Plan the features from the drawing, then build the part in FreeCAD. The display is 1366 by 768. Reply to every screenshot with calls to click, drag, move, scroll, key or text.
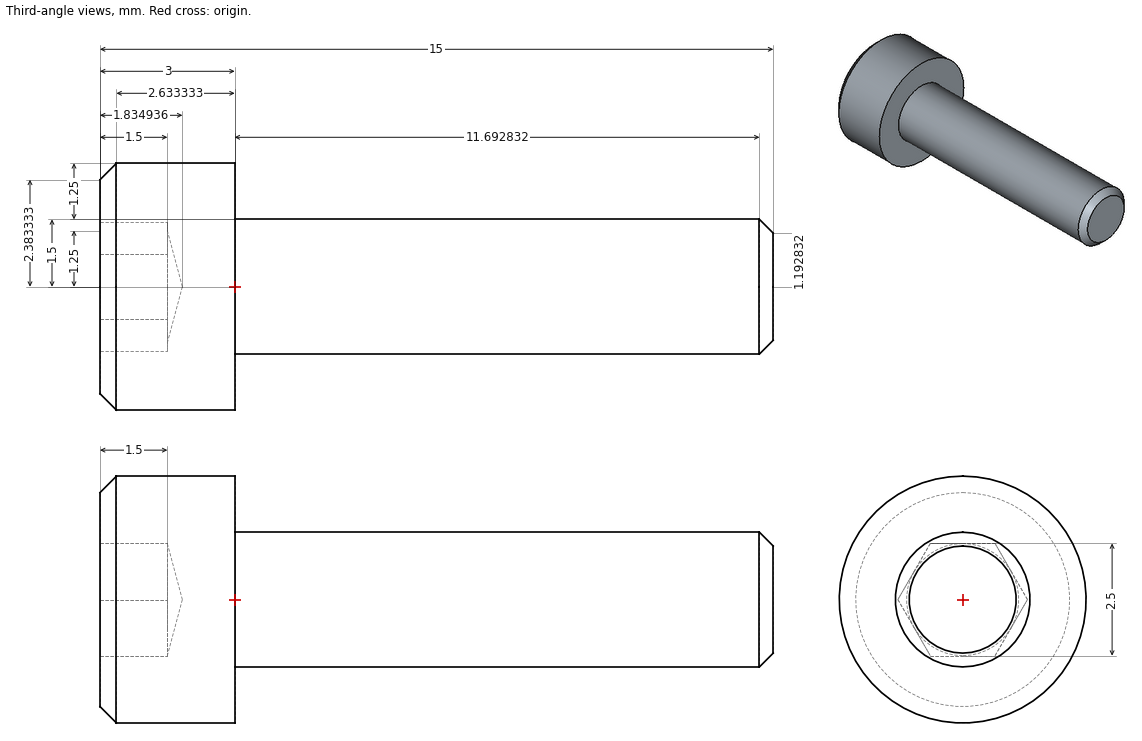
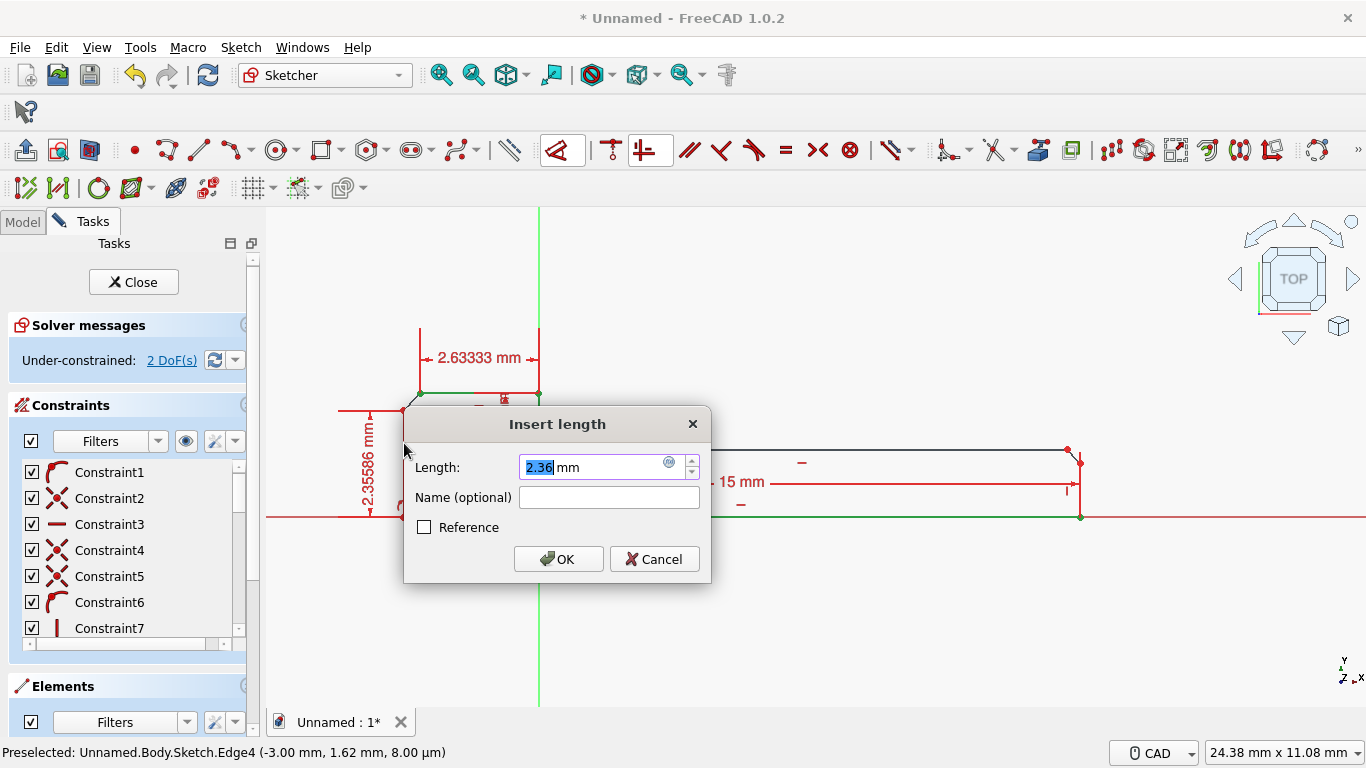
text(2.383333)
key(Return)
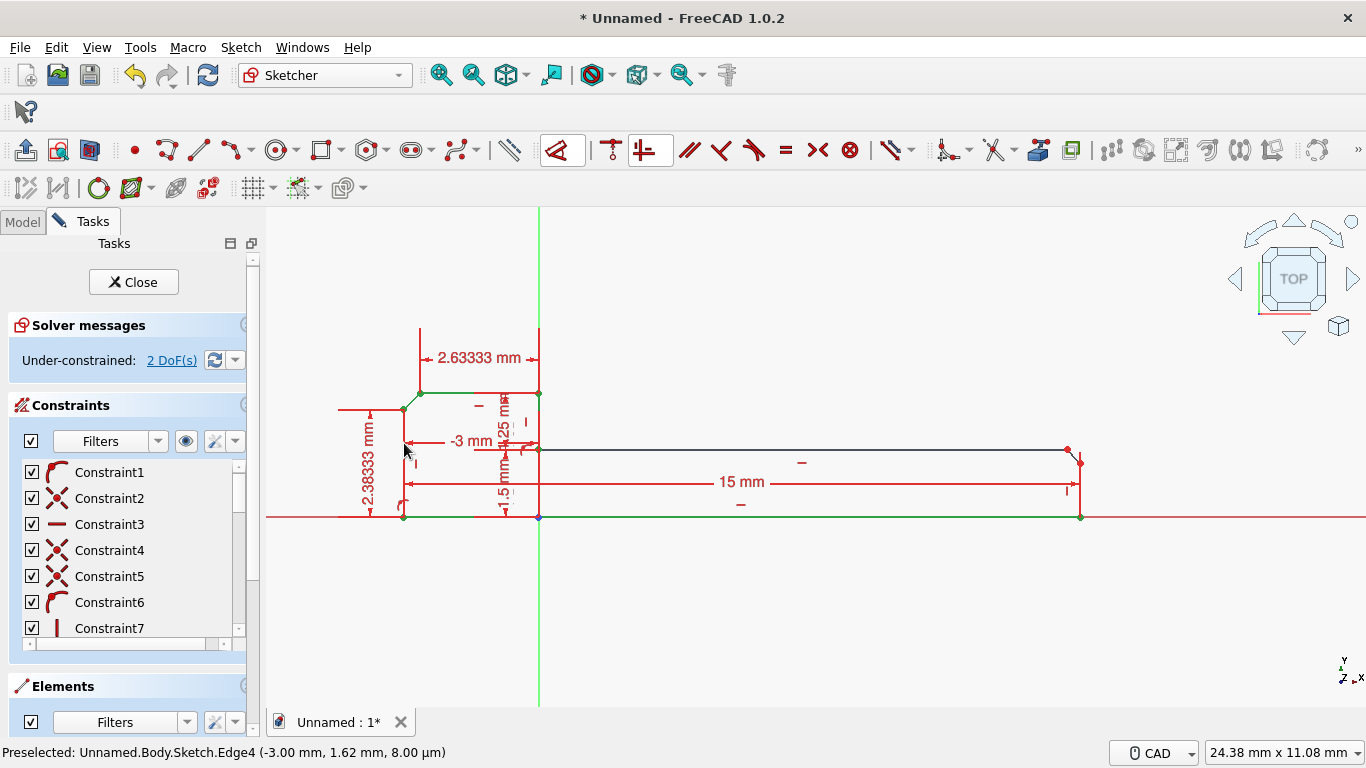
click(1080, 501)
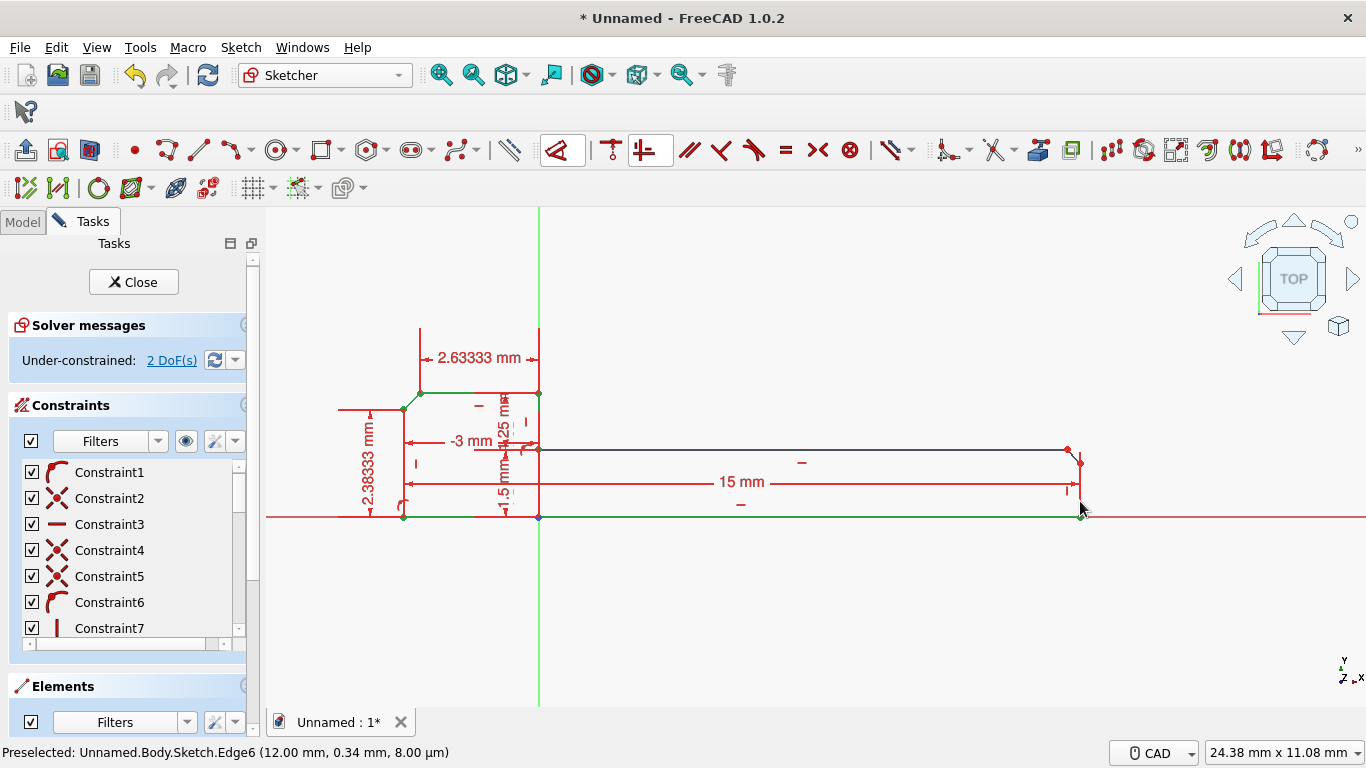
click(580, 150)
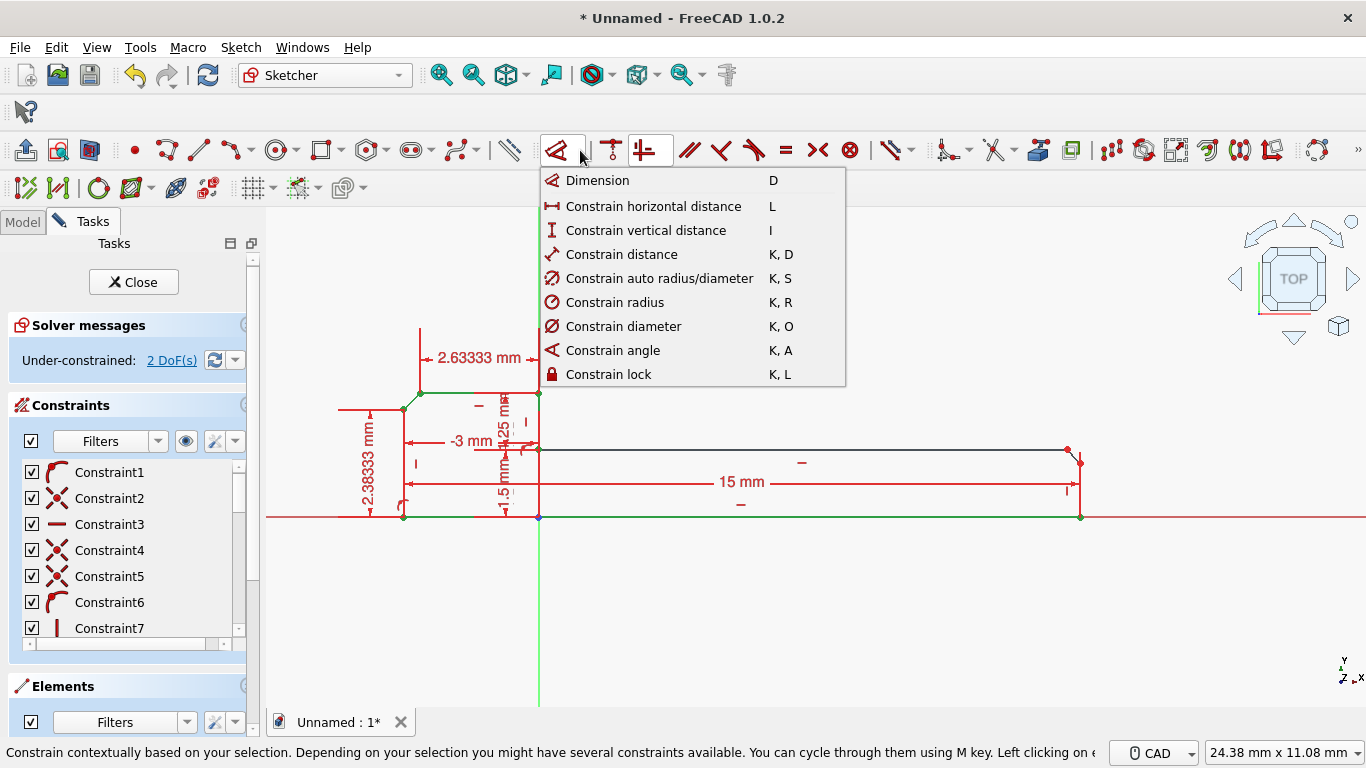
click(693, 230)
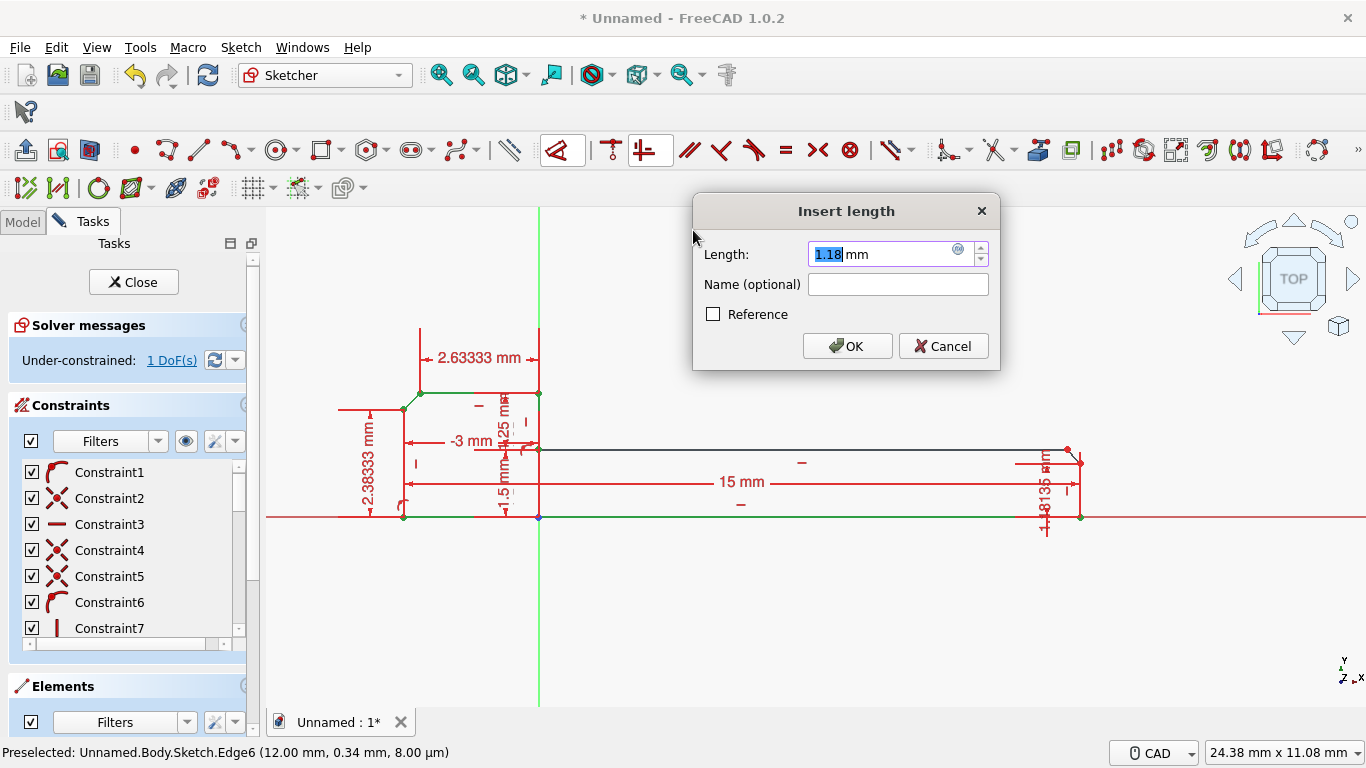
text(1.192832)
key(Return)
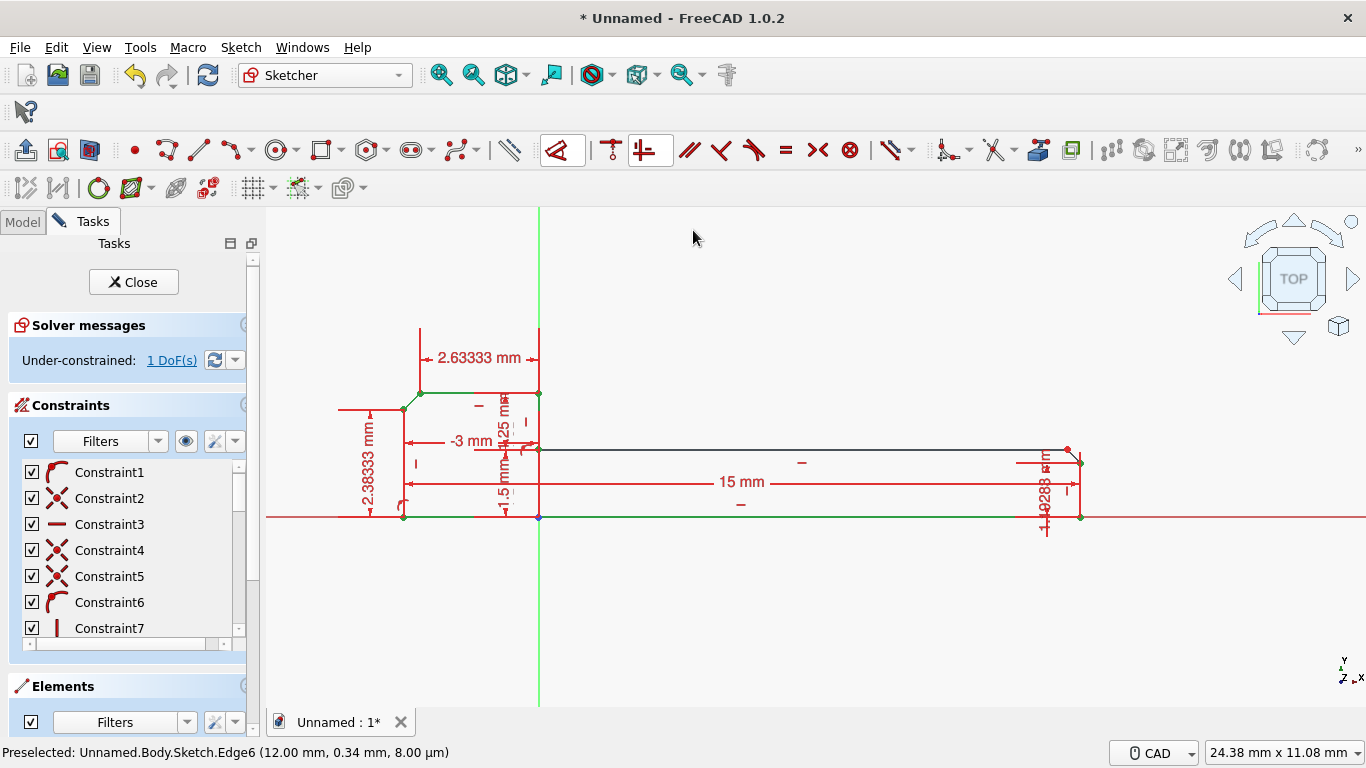
click(909, 450)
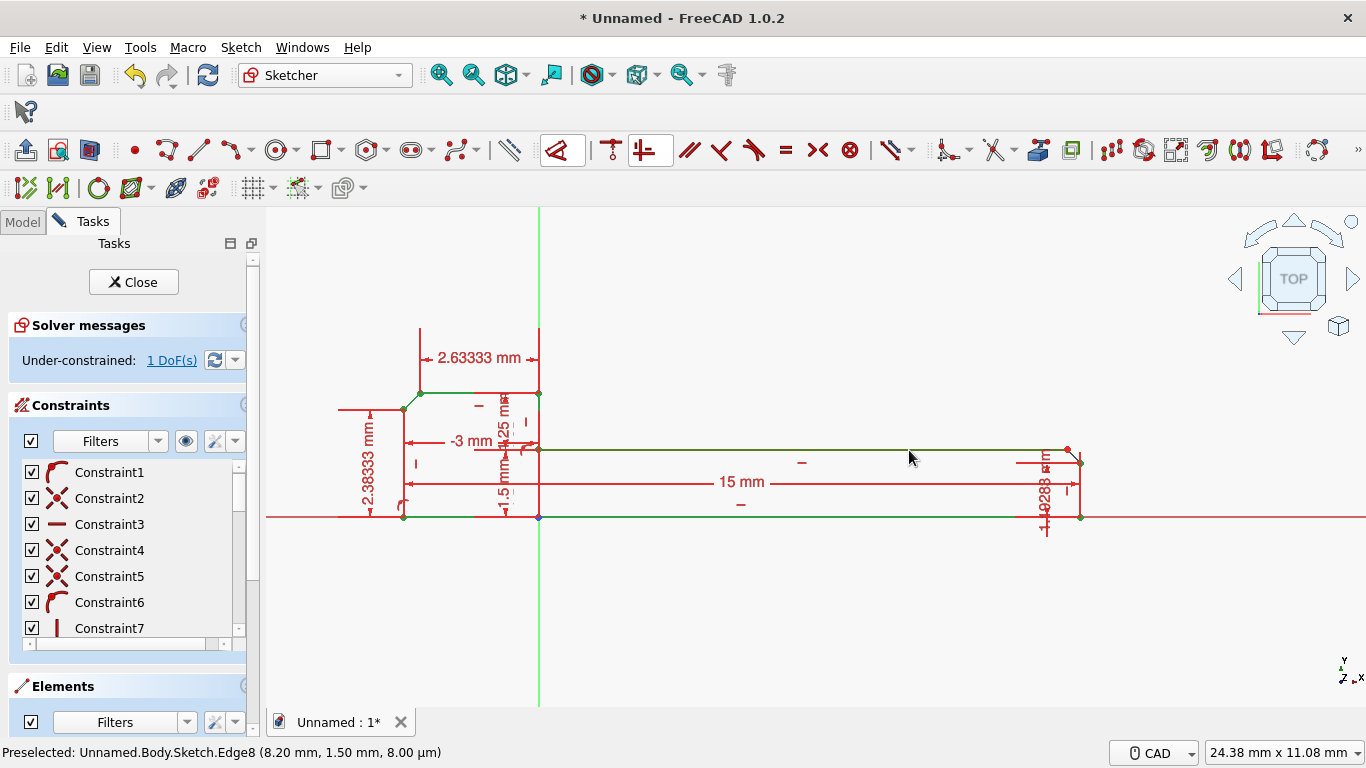
click(580, 150)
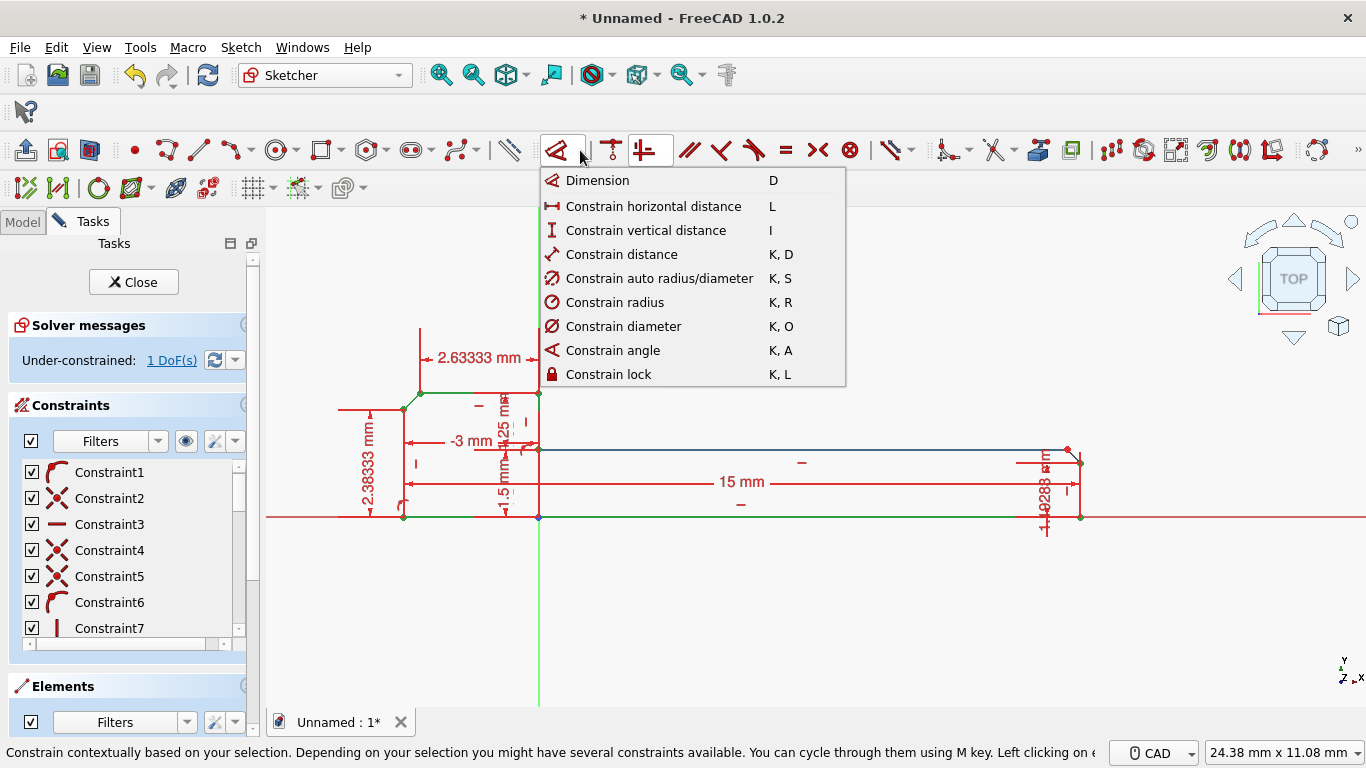
click(693, 206)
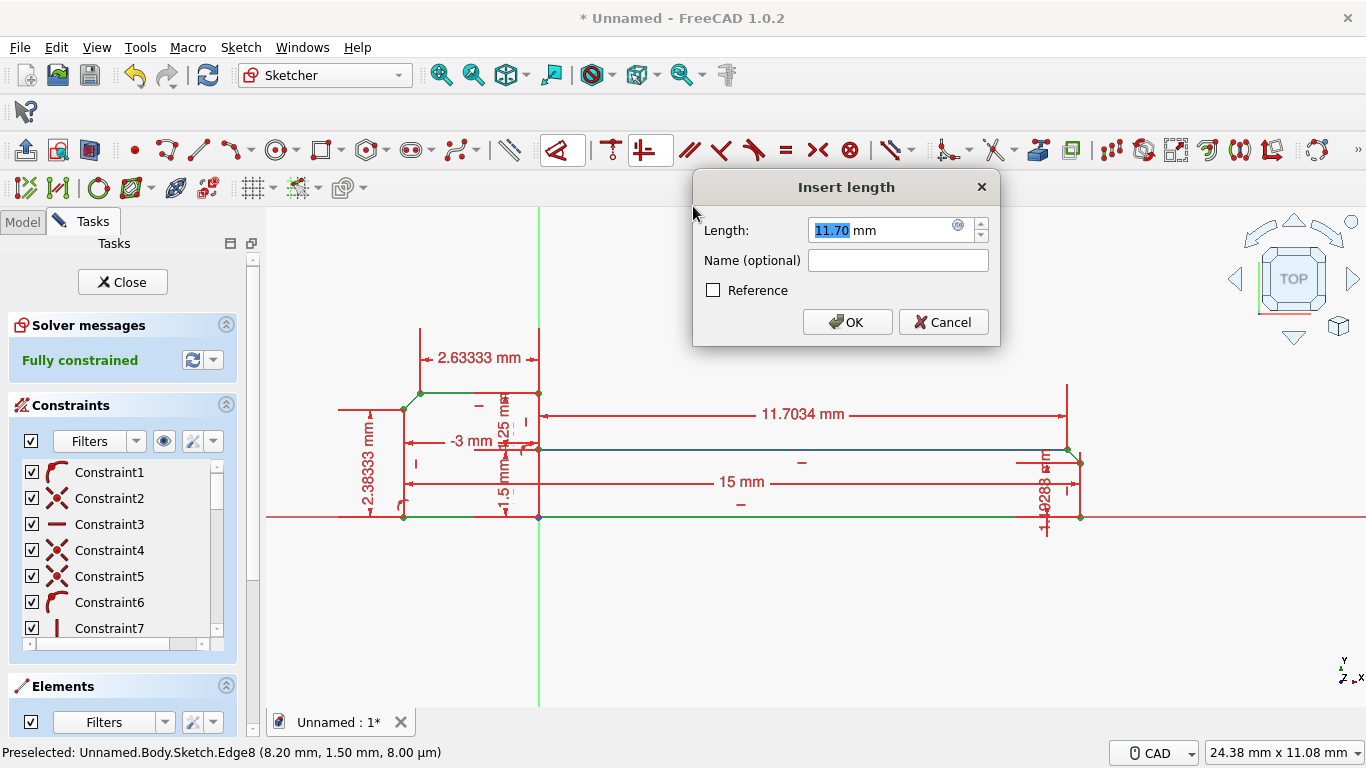
text(11.692832)
key(Return)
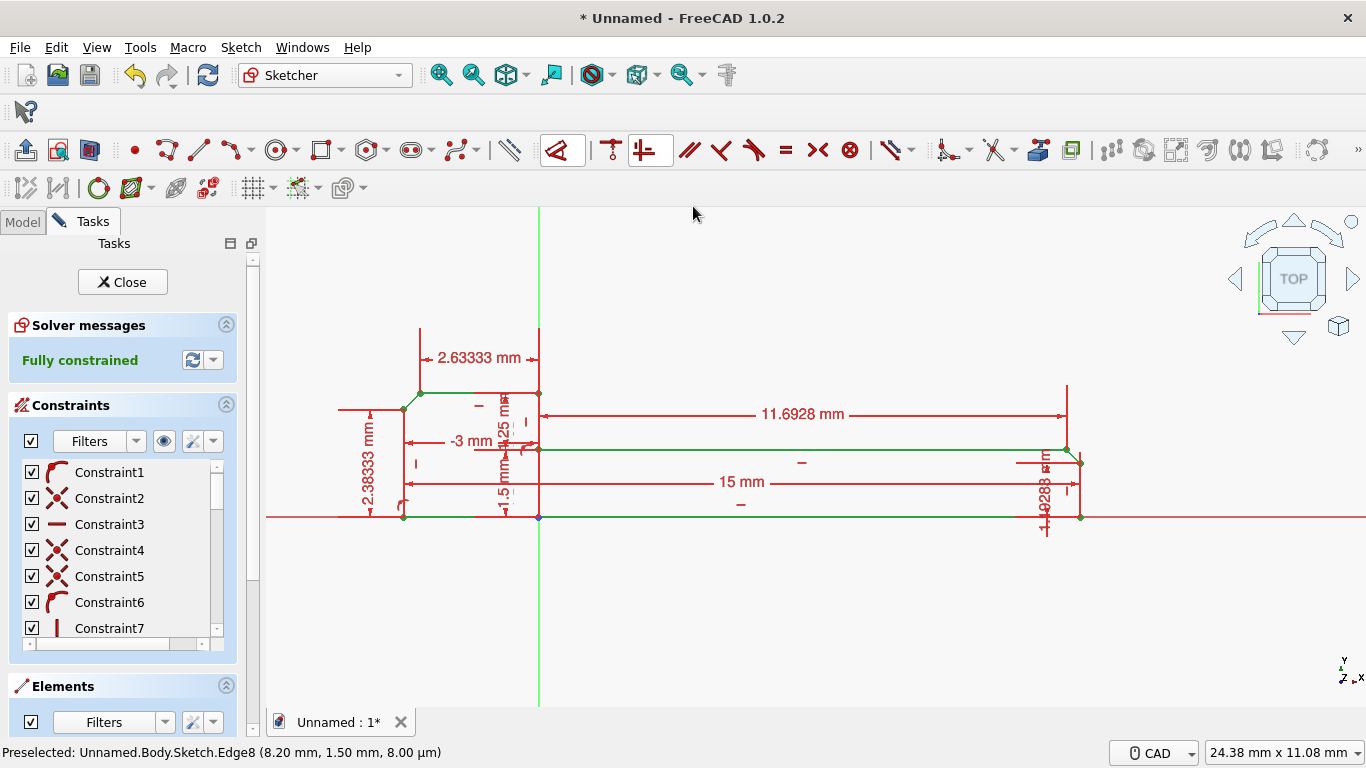
click(123, 282)